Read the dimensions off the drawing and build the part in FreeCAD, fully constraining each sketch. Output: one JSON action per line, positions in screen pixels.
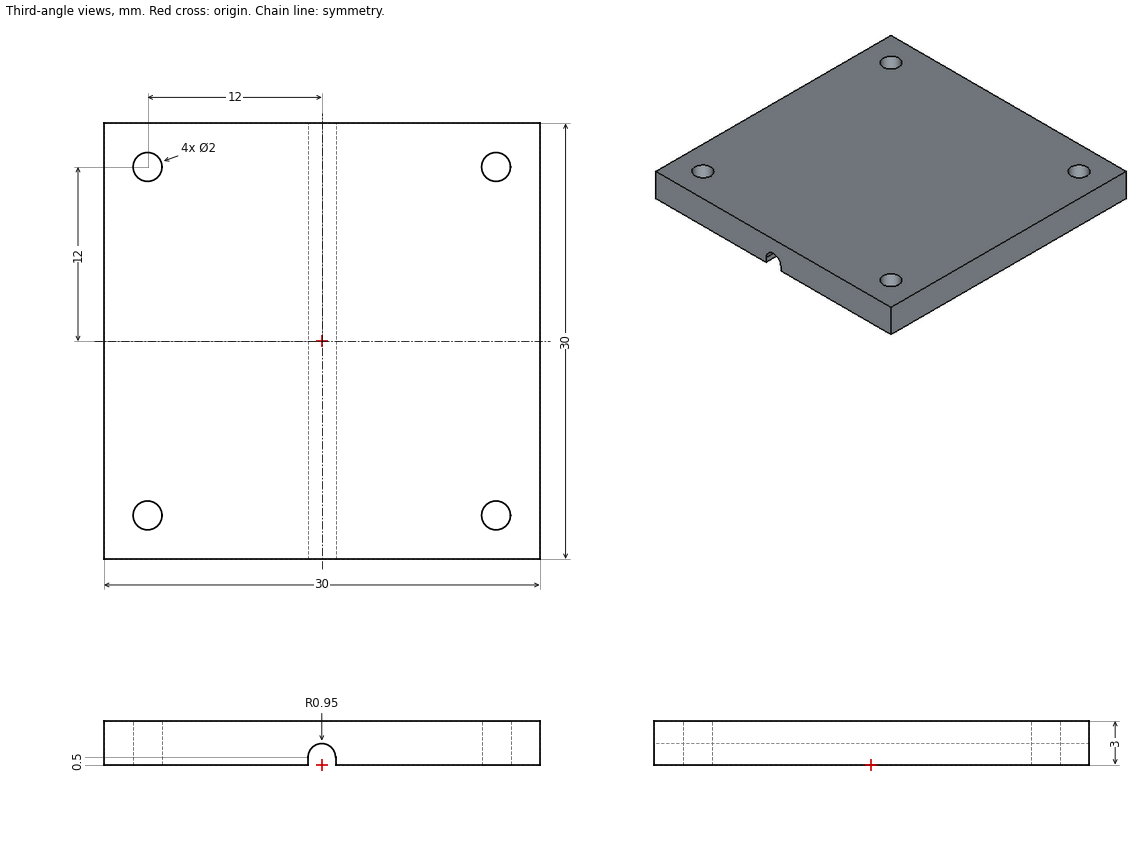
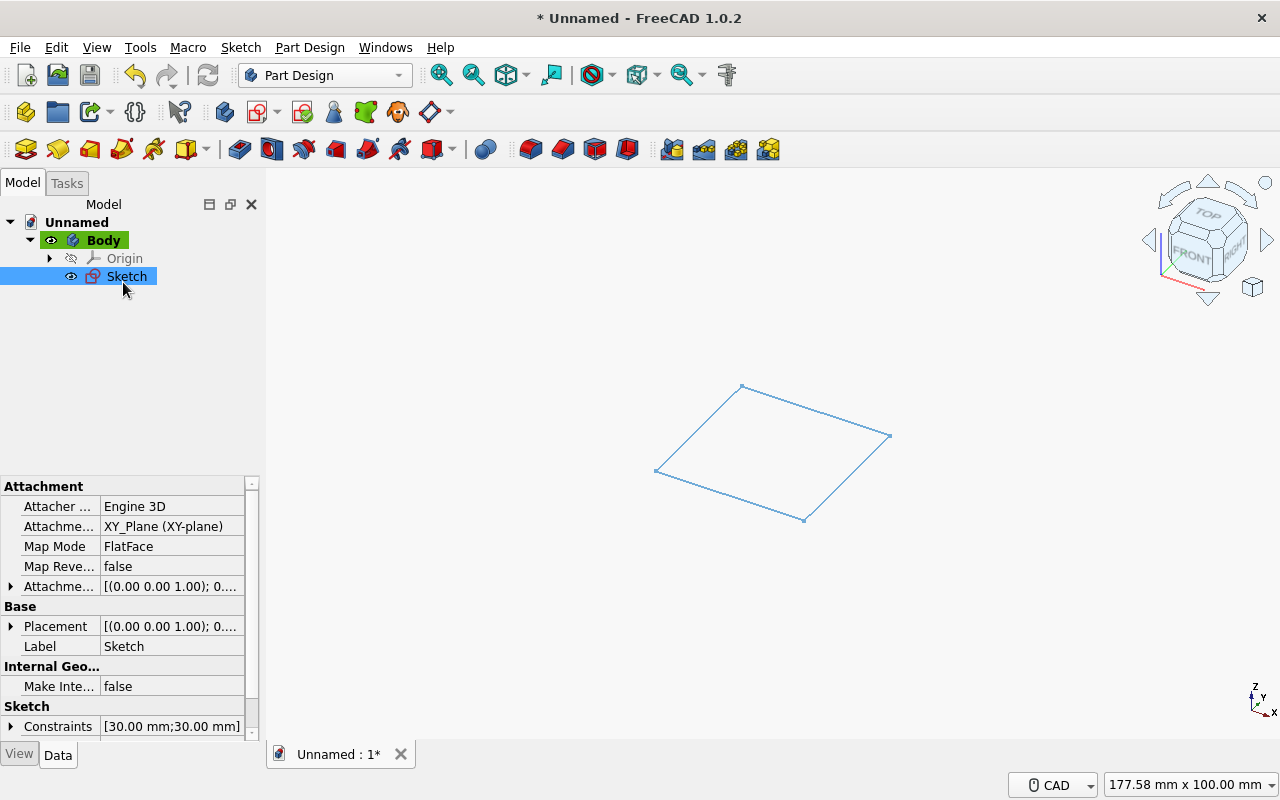
{"action": "left_click", "coordinate": [26, 150]}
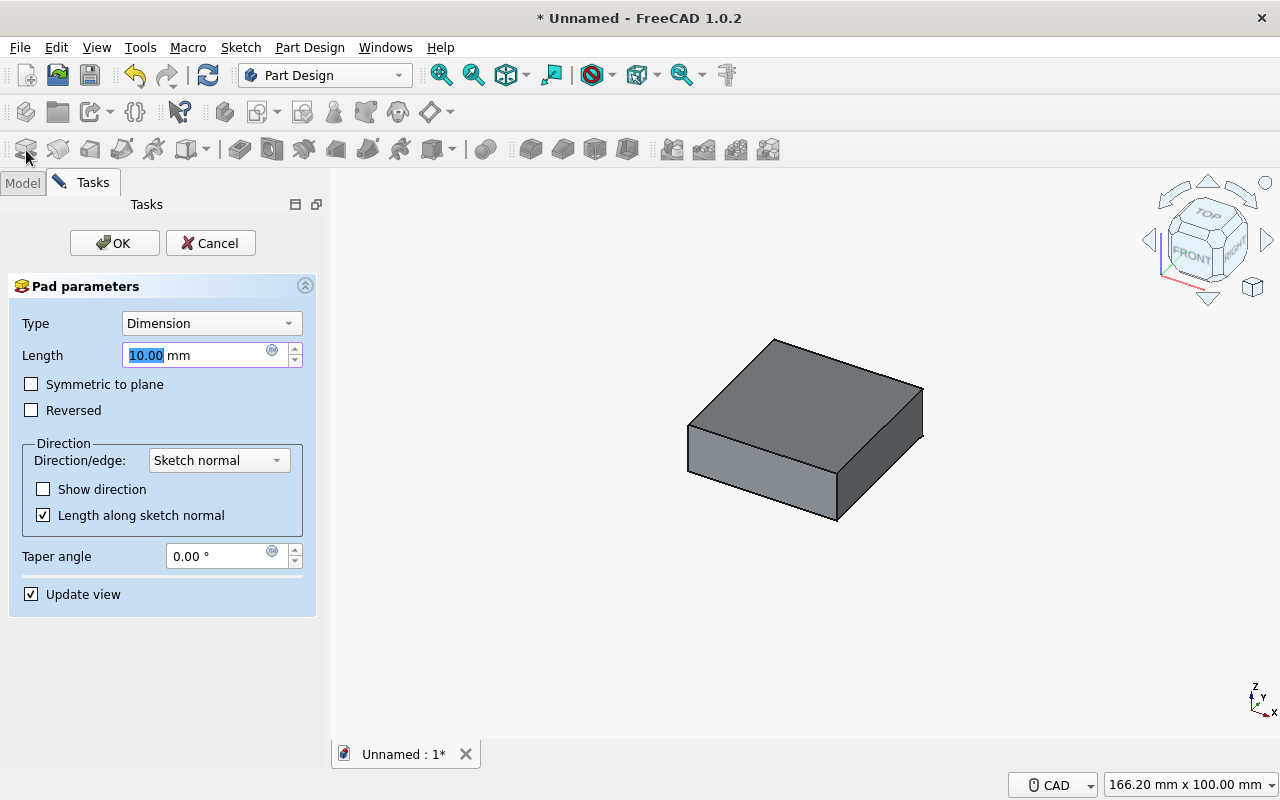
{"action": "type", "text": "3"}
{"action": "key", "text": "Tab"}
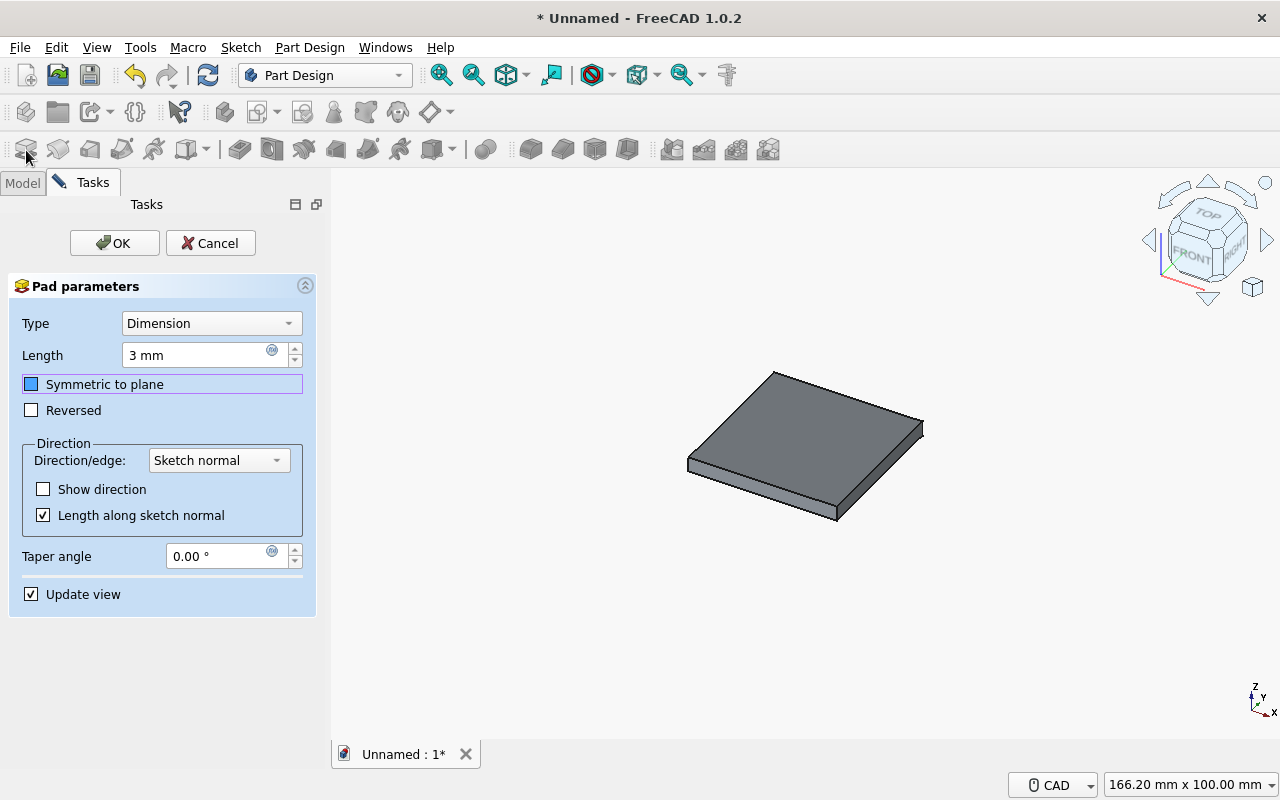
{"action": "left_click", "coordinate": [115, 243]}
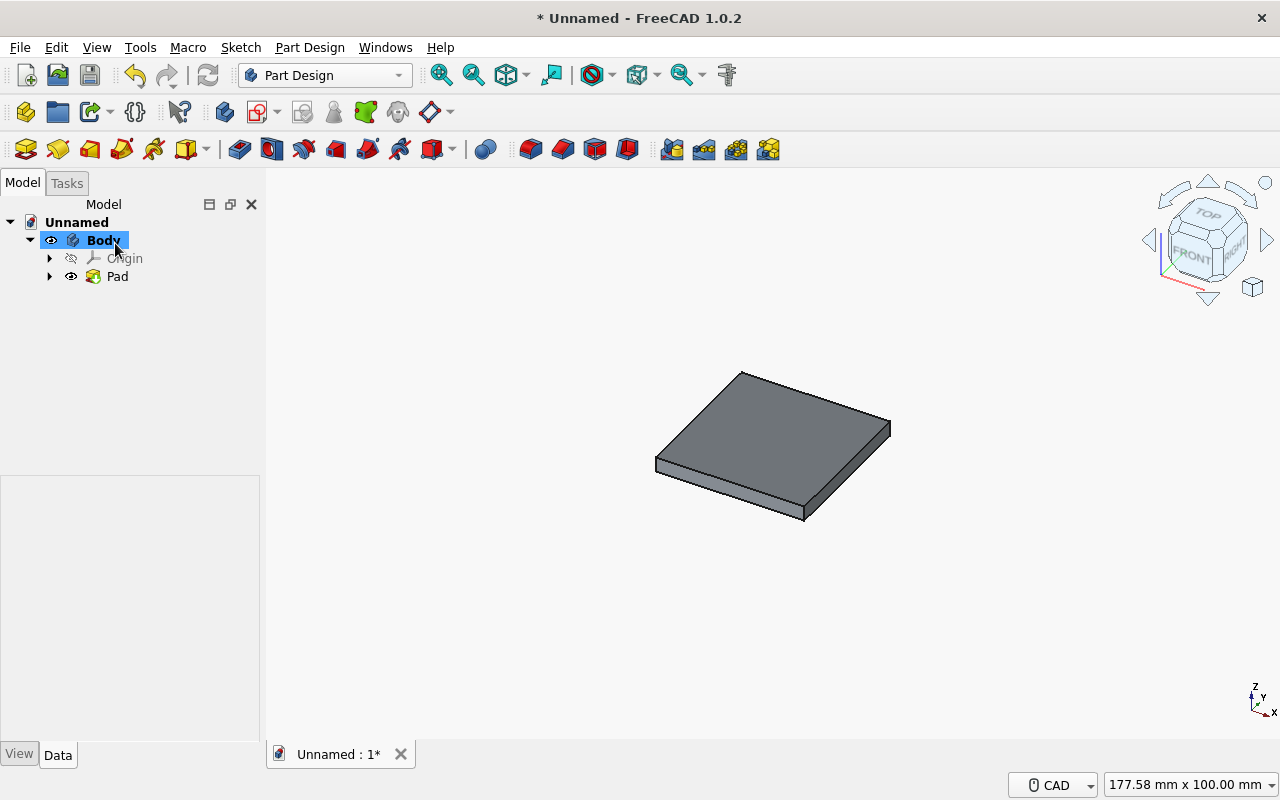
{"action": "key", "text": "v f"}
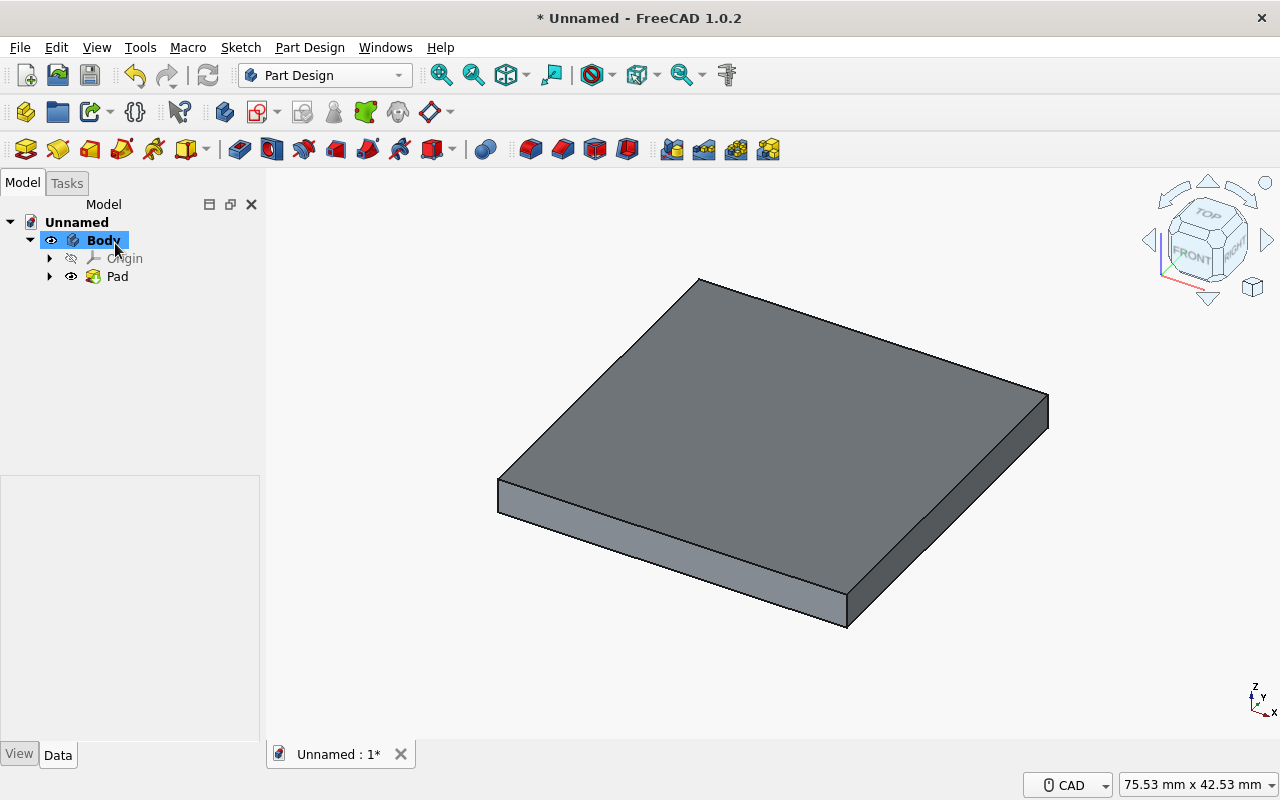
{"action": "left_click", "coordinate": [773, 436]}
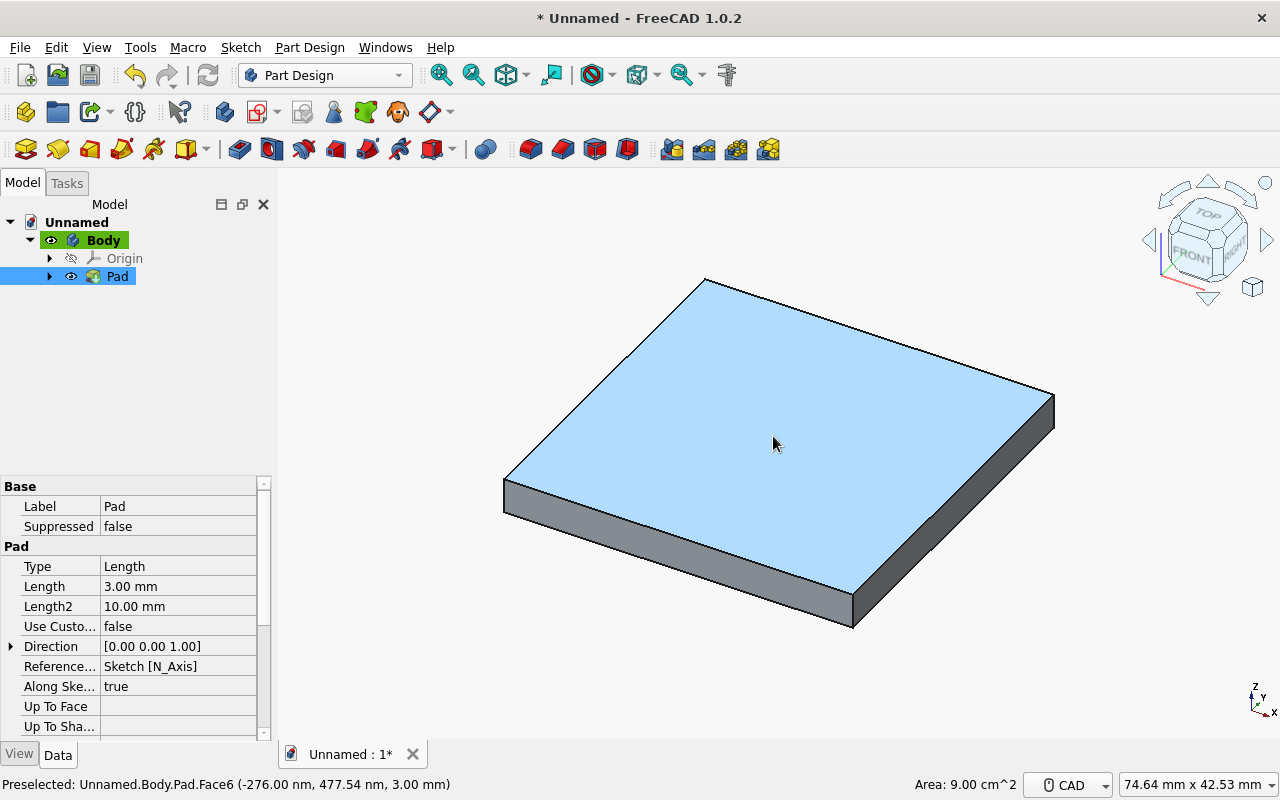
{"action": "left_click", "coordinate": [258, 112]}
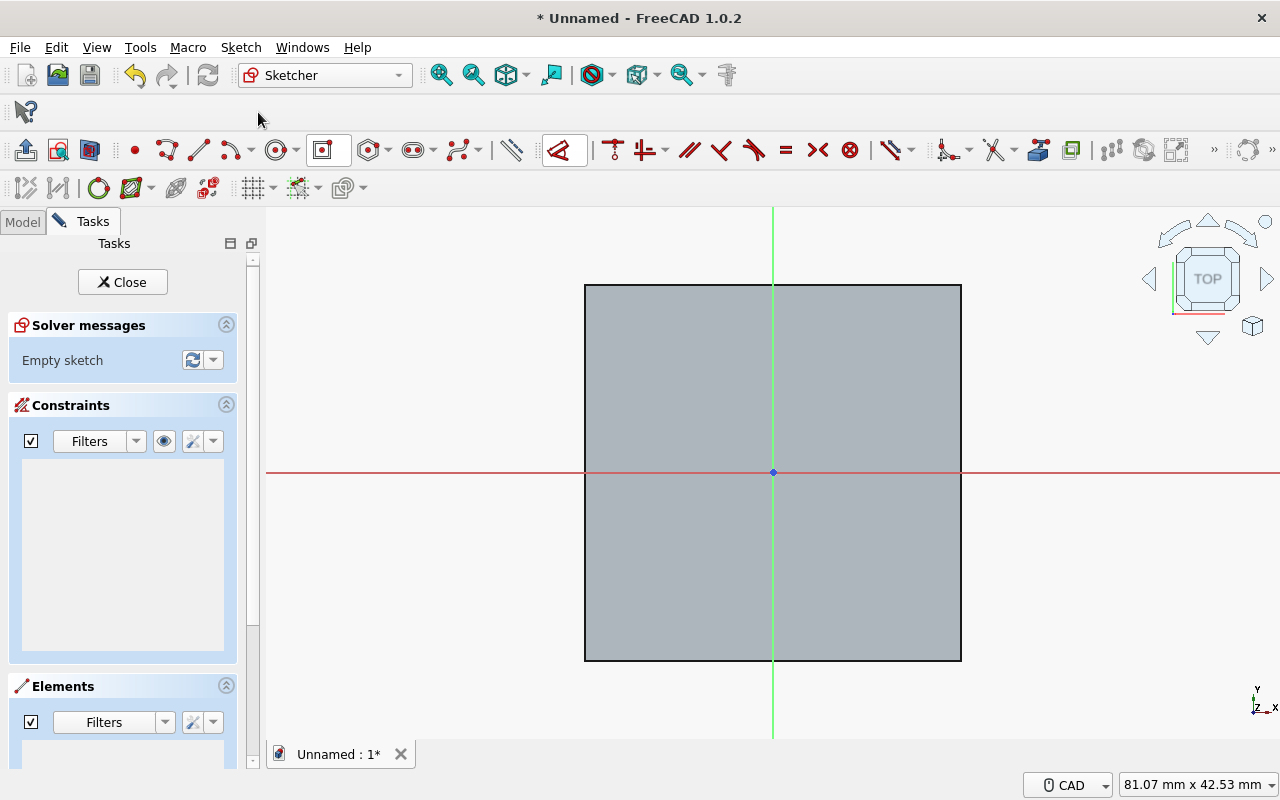
{"action": "key", "text": "g c"}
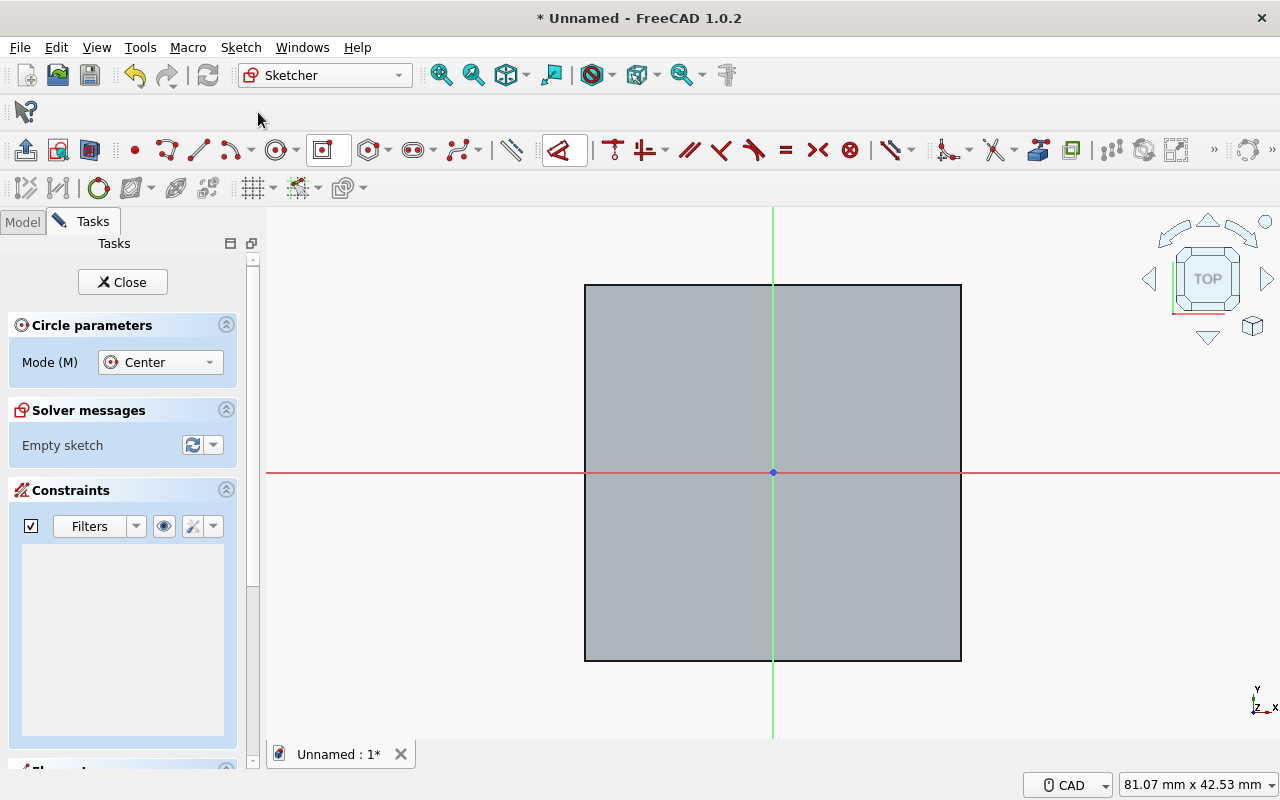
{"action": "scroll", "coordinate": [623, 323], "scroll_direction": "up", "scroll_amount": 3}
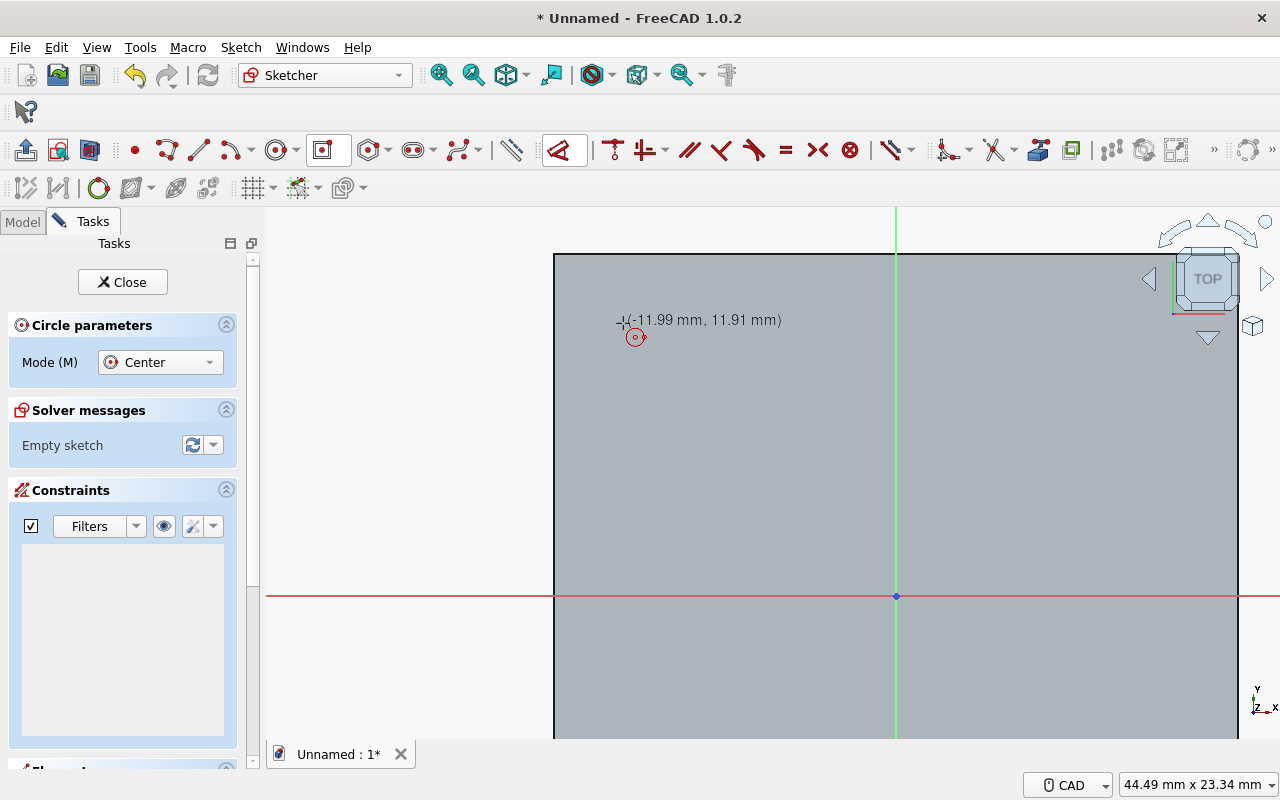
{"action": "left_click", "coordinate": [623, 323]}
{"action": "mouse_move", "coordinate": [639, 307]}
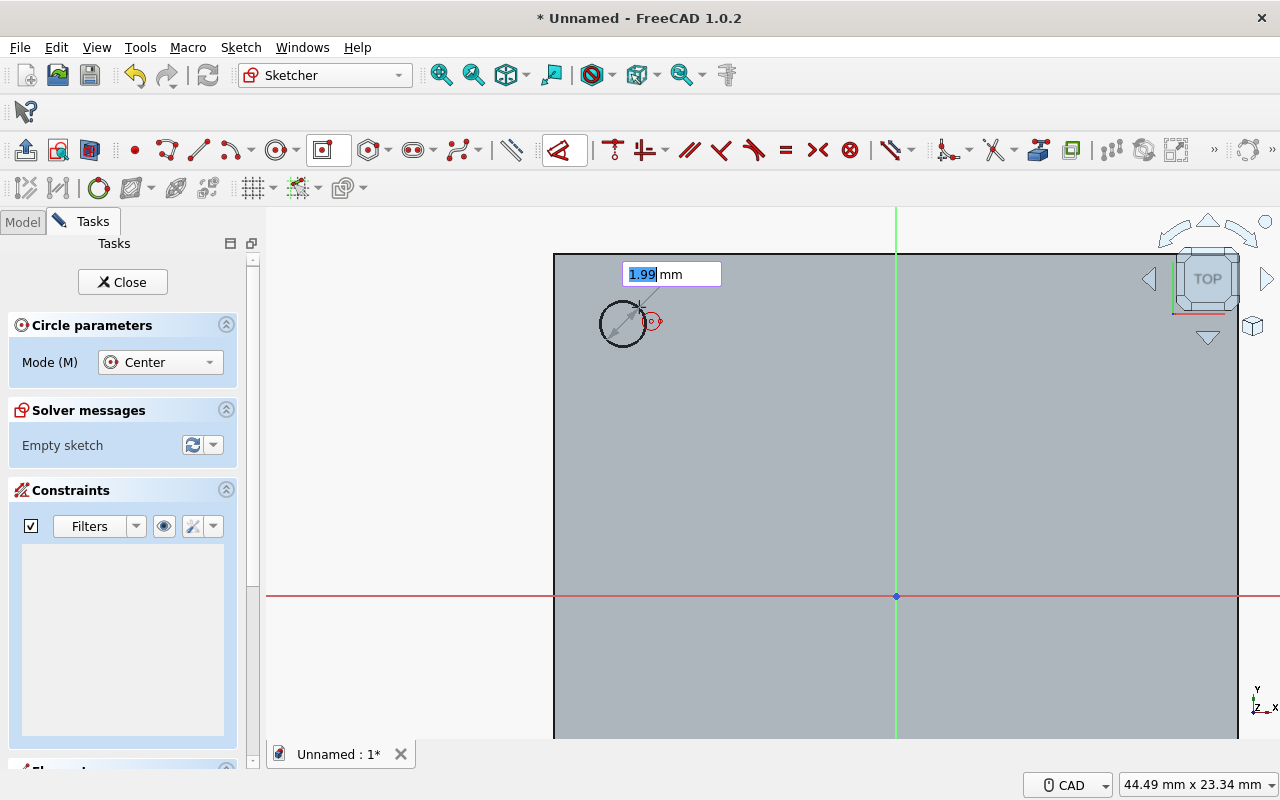
{"action": "type", "text": "2"}
{"action": "key", "text": "Return"}